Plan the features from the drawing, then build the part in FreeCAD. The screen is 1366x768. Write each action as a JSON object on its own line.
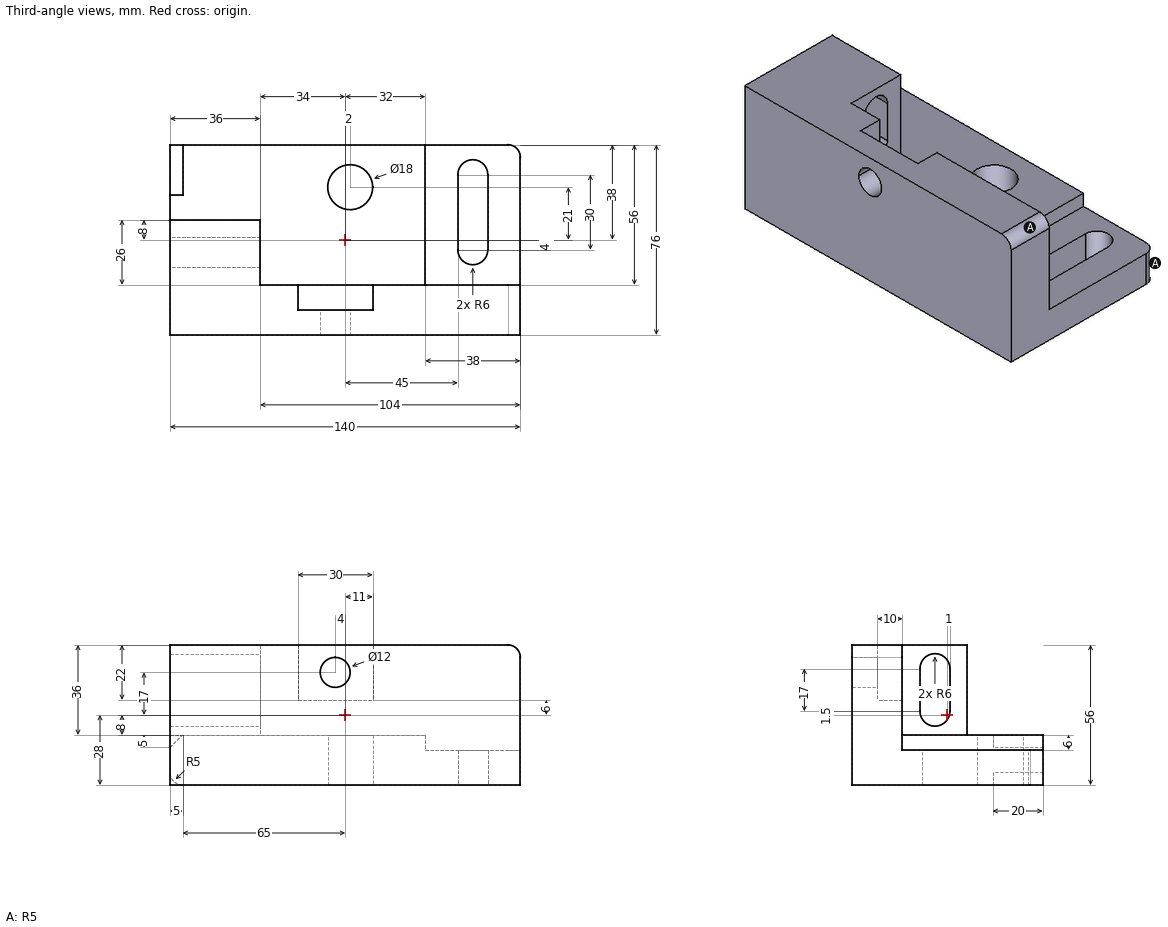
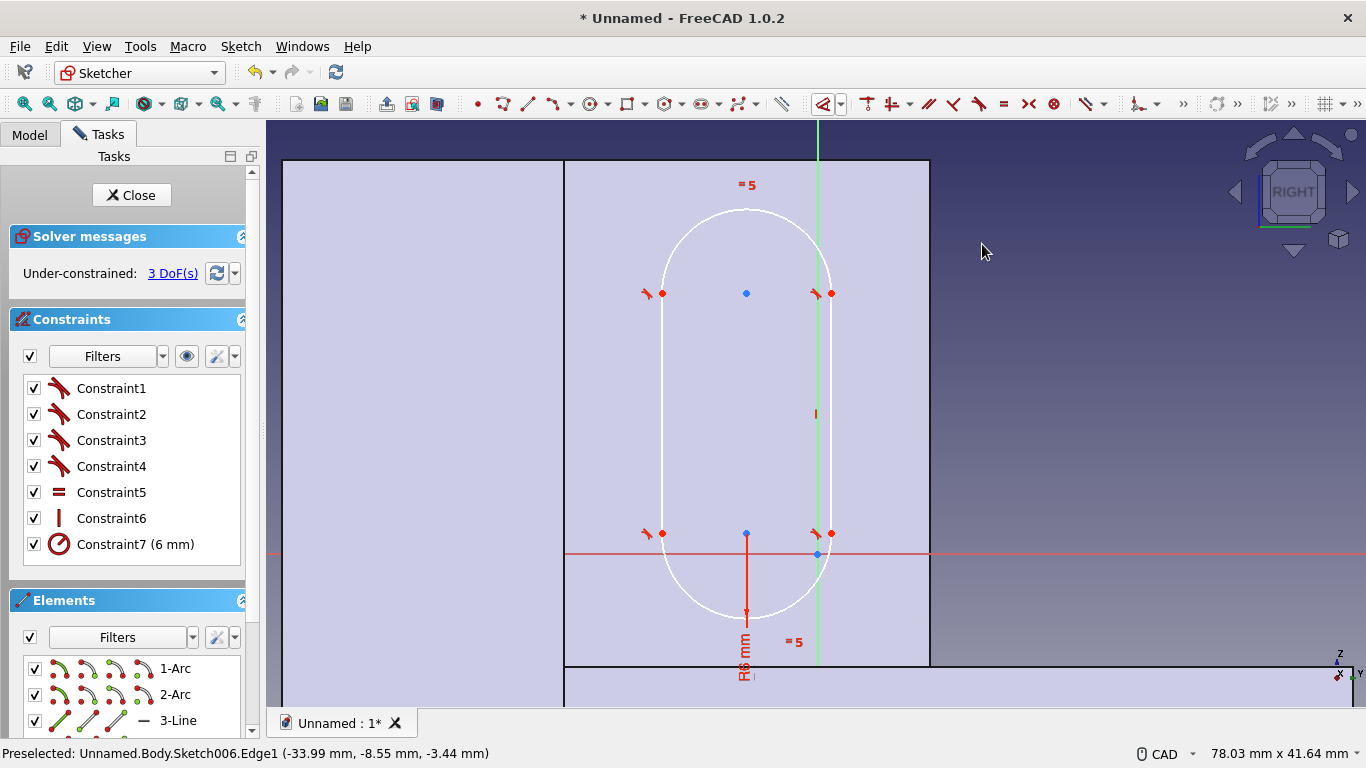
{"action": "left_click", "coordinate": [662, 462]}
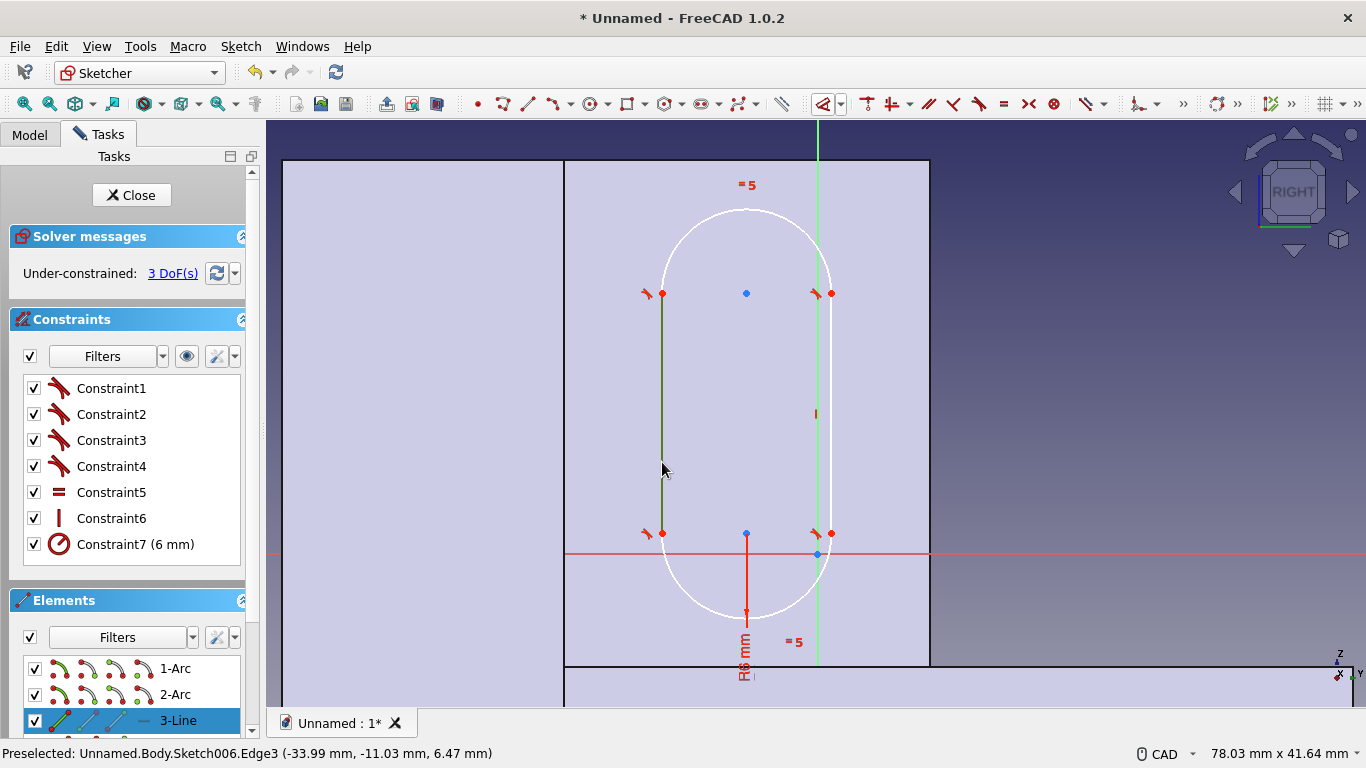
{"action": "key", "text": "i"}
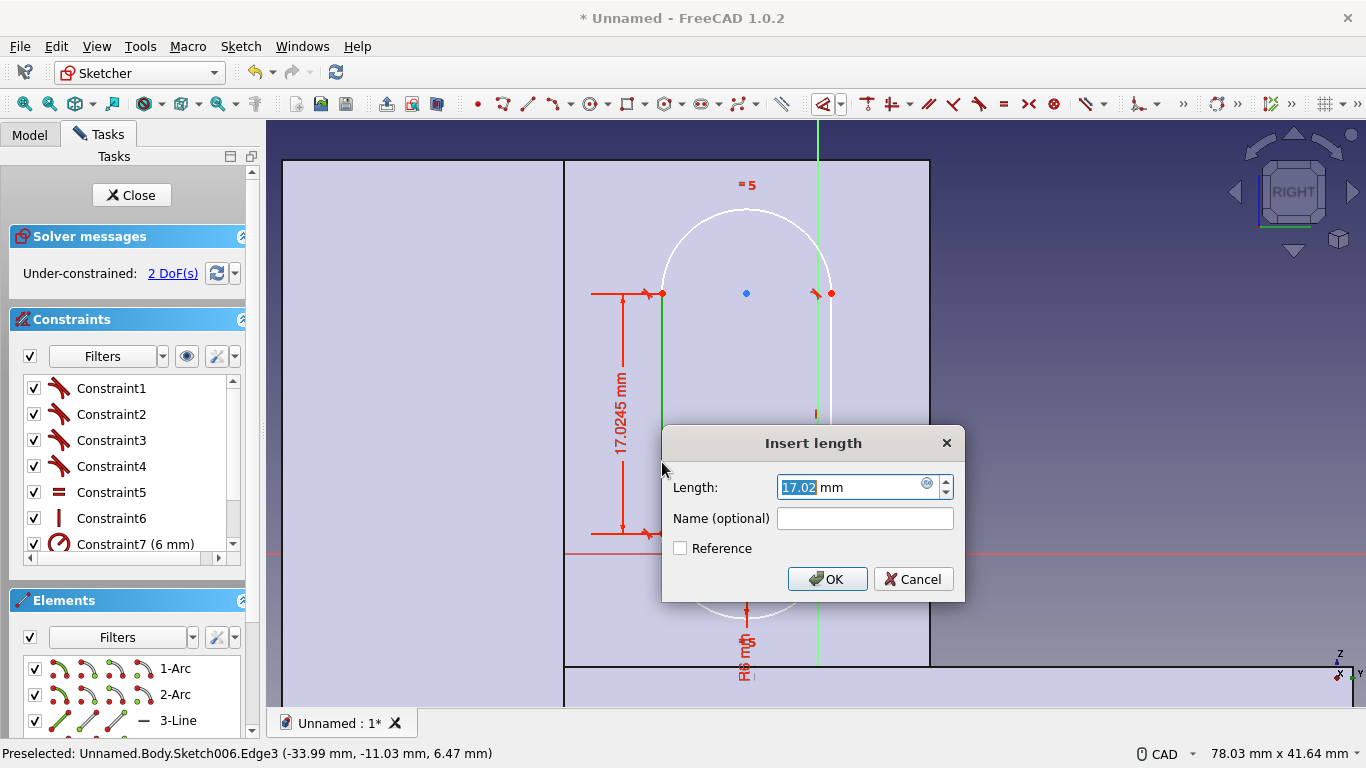
{"action": "type", "text": "17"}
{"action": "key", "text": "Return"}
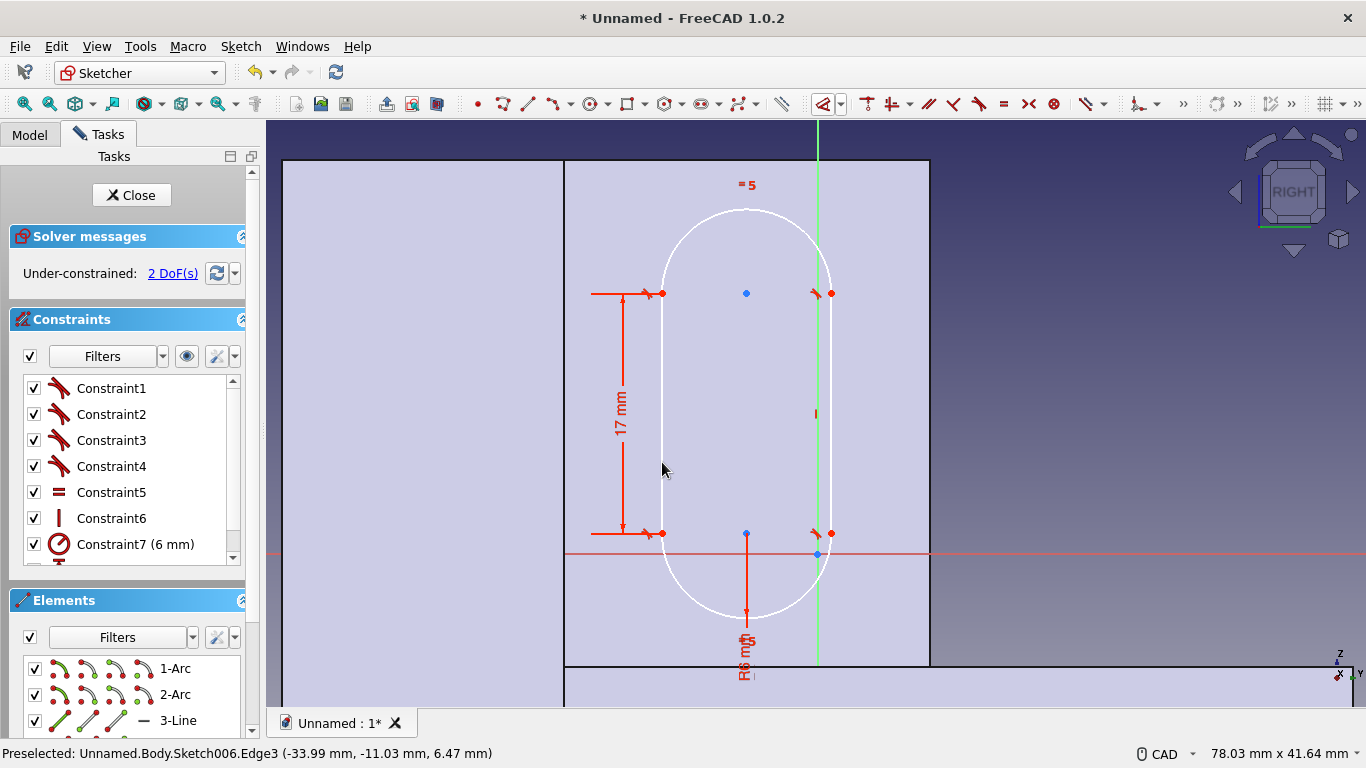
{"action": "scroll", "coordinate": [831, 534], "scroll_direction": "up", "scroll_amount": 6}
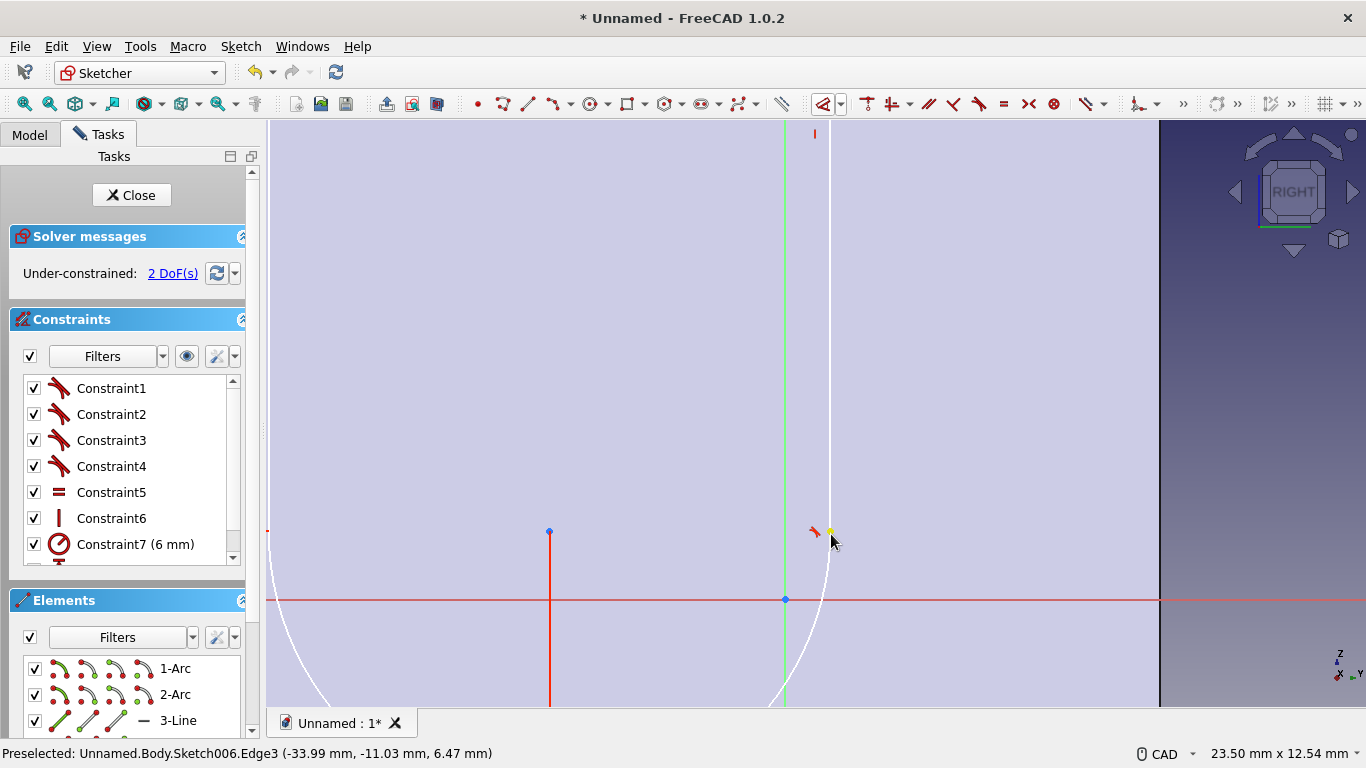
{"action": "left_click", "coordinate": [830, 531]}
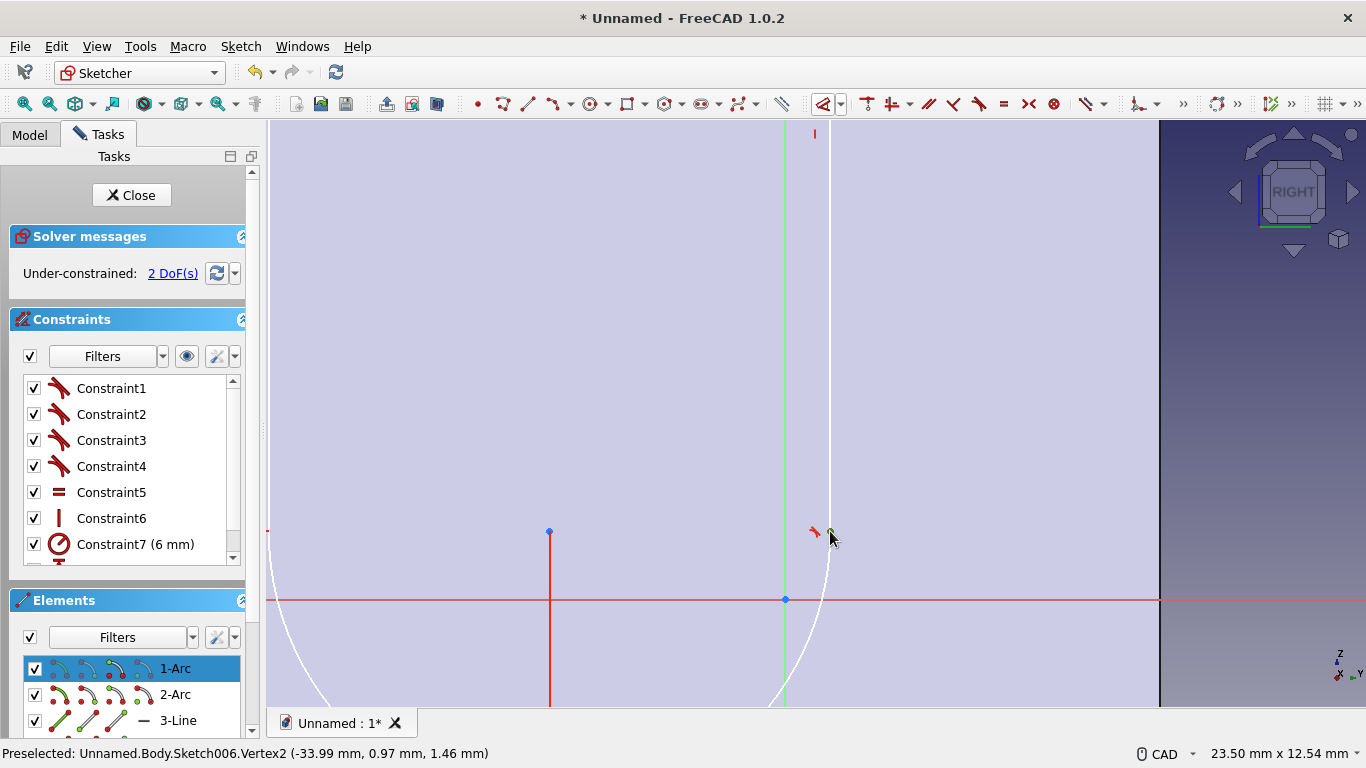
{"action": "left_click", "coordinate": [840, 104]}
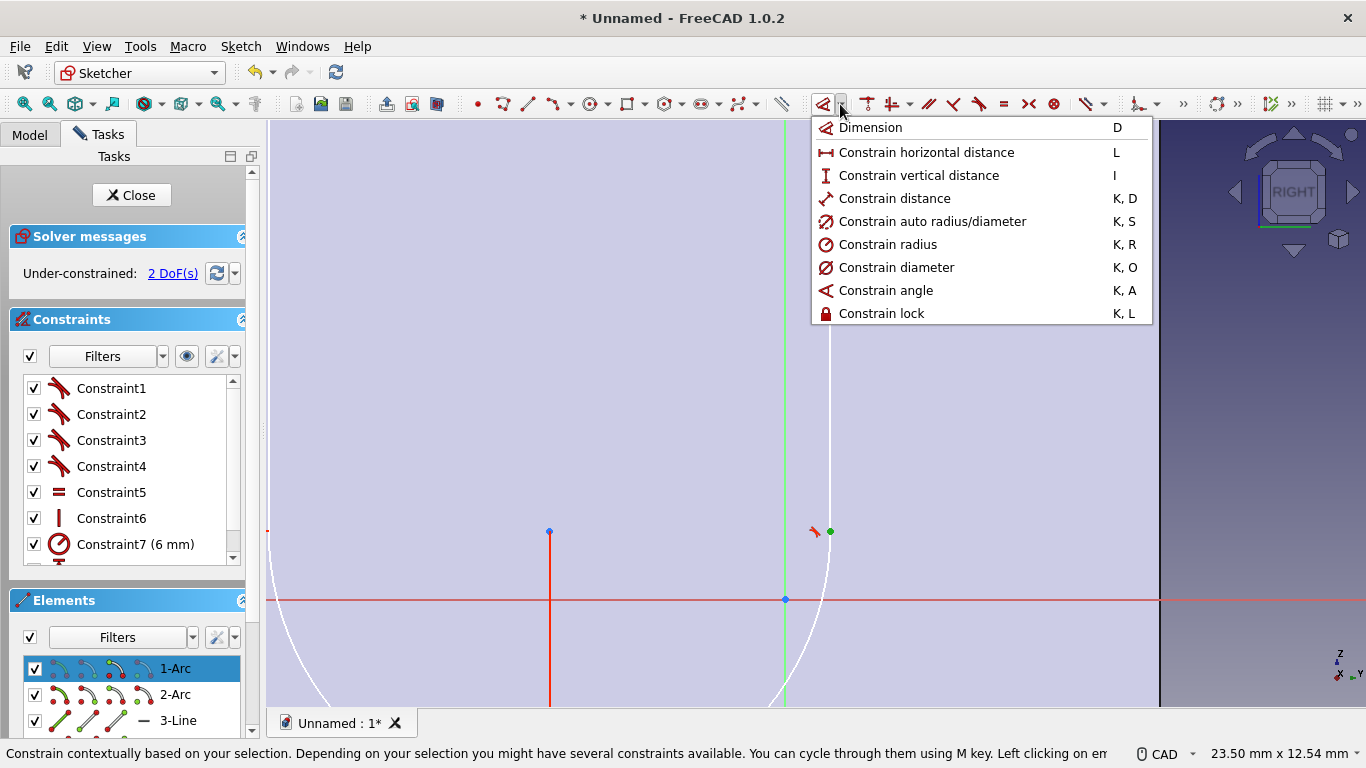
{"action": "left_click", "coordinate": [982, 152]}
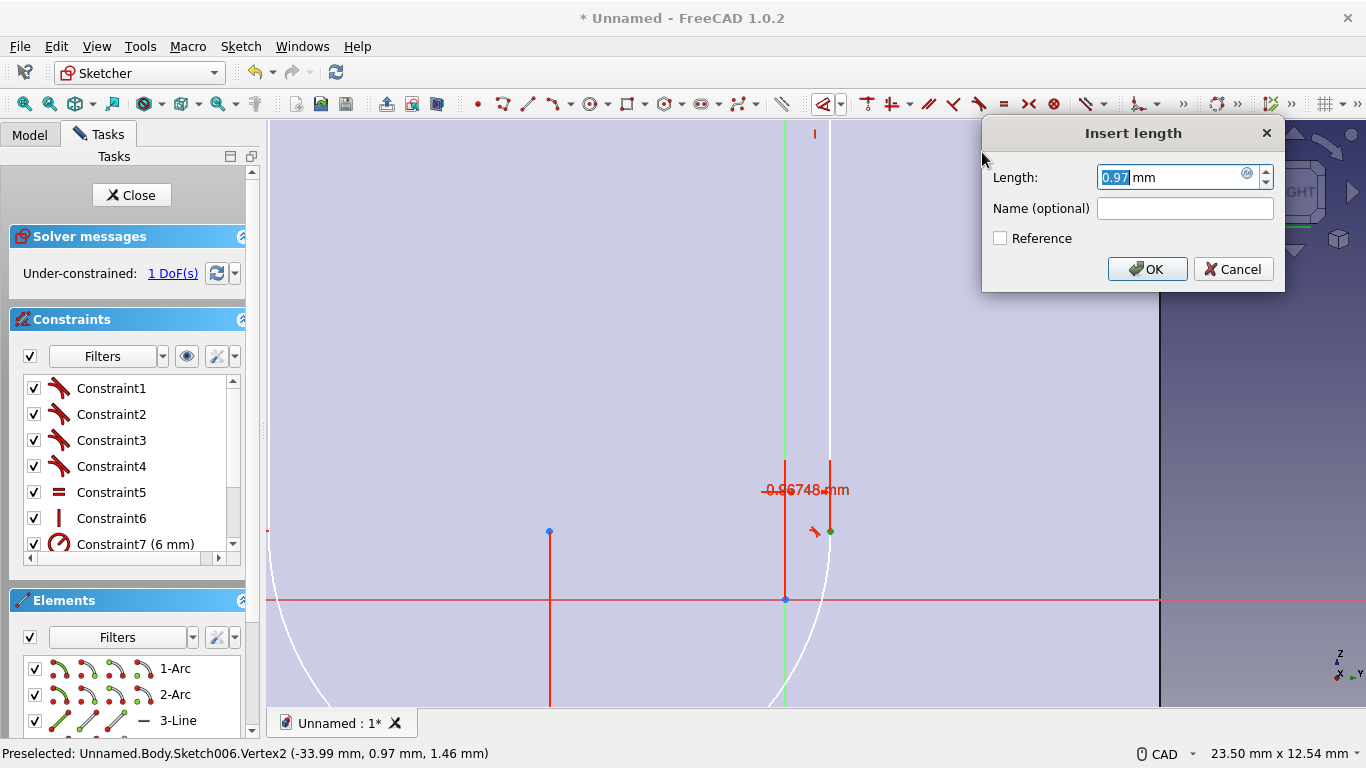
{"action": "type", "text": "1"}
{"action": "key", "text": "Return"}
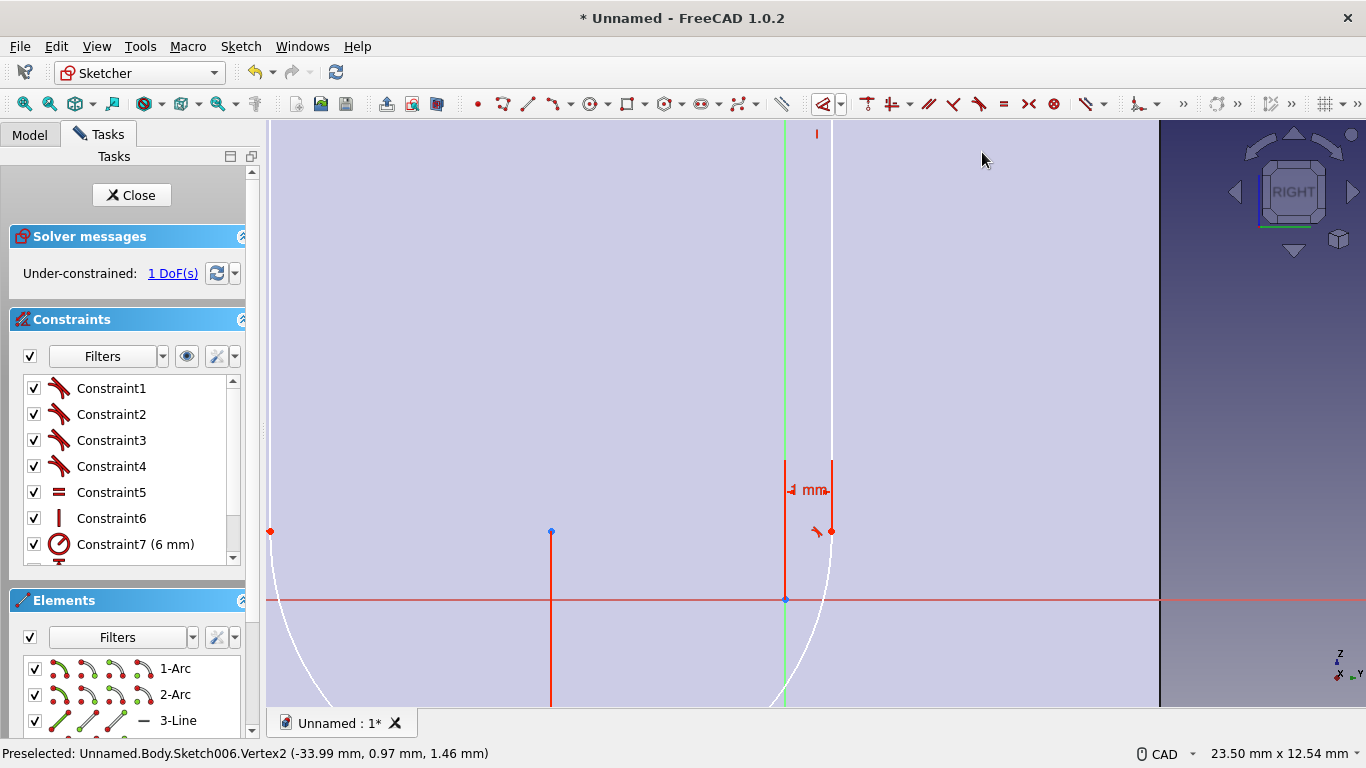
{"action": "scroll", "coordinate": [832, 535], "scroll_direction": "down", "scroll_amount": 6}